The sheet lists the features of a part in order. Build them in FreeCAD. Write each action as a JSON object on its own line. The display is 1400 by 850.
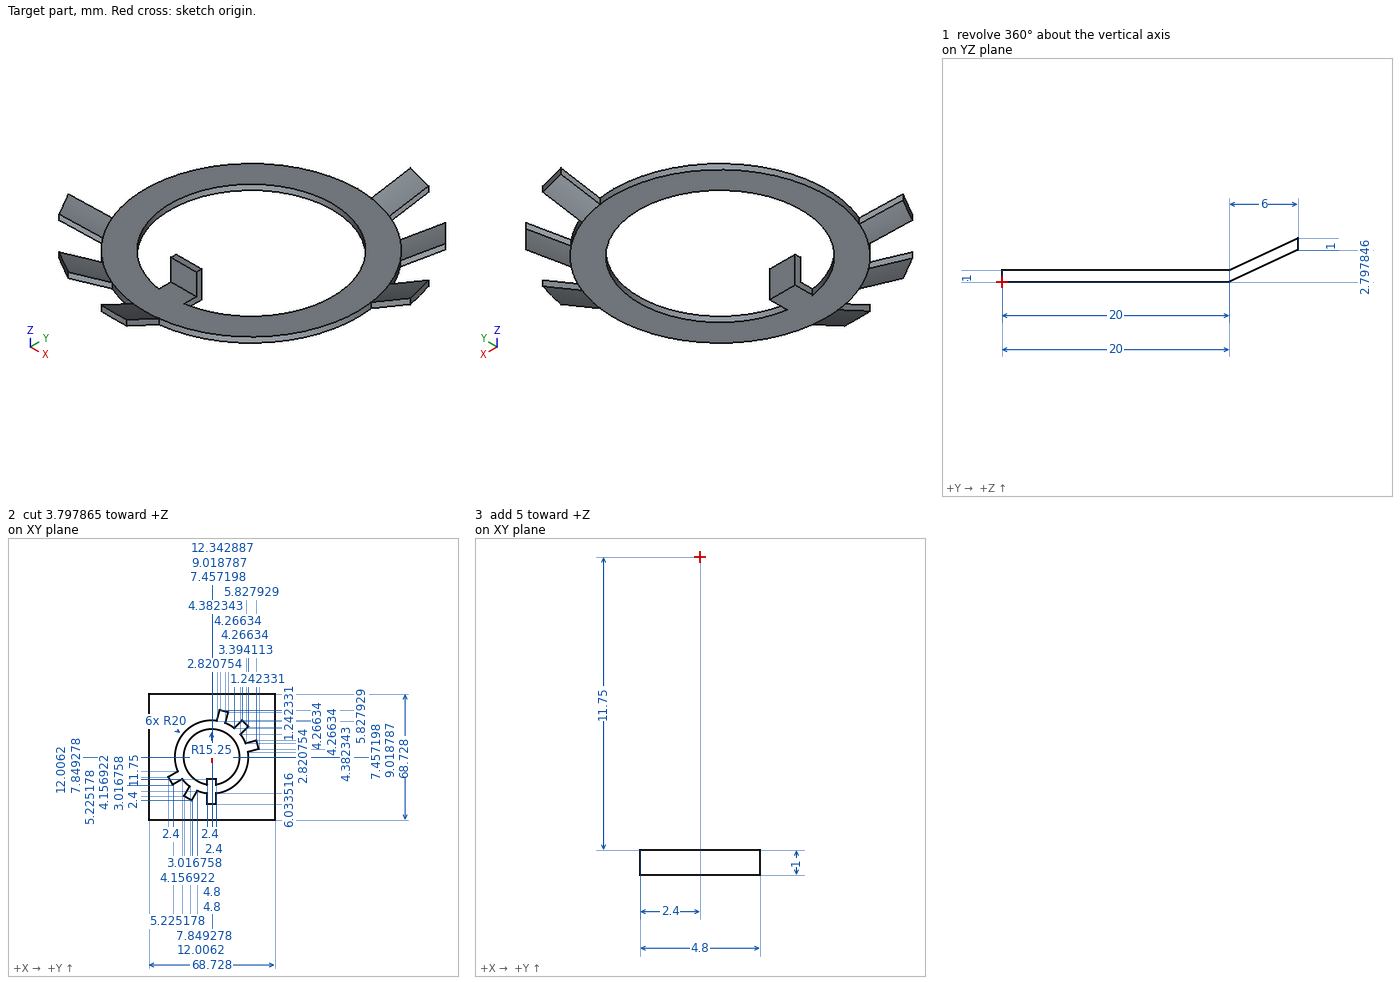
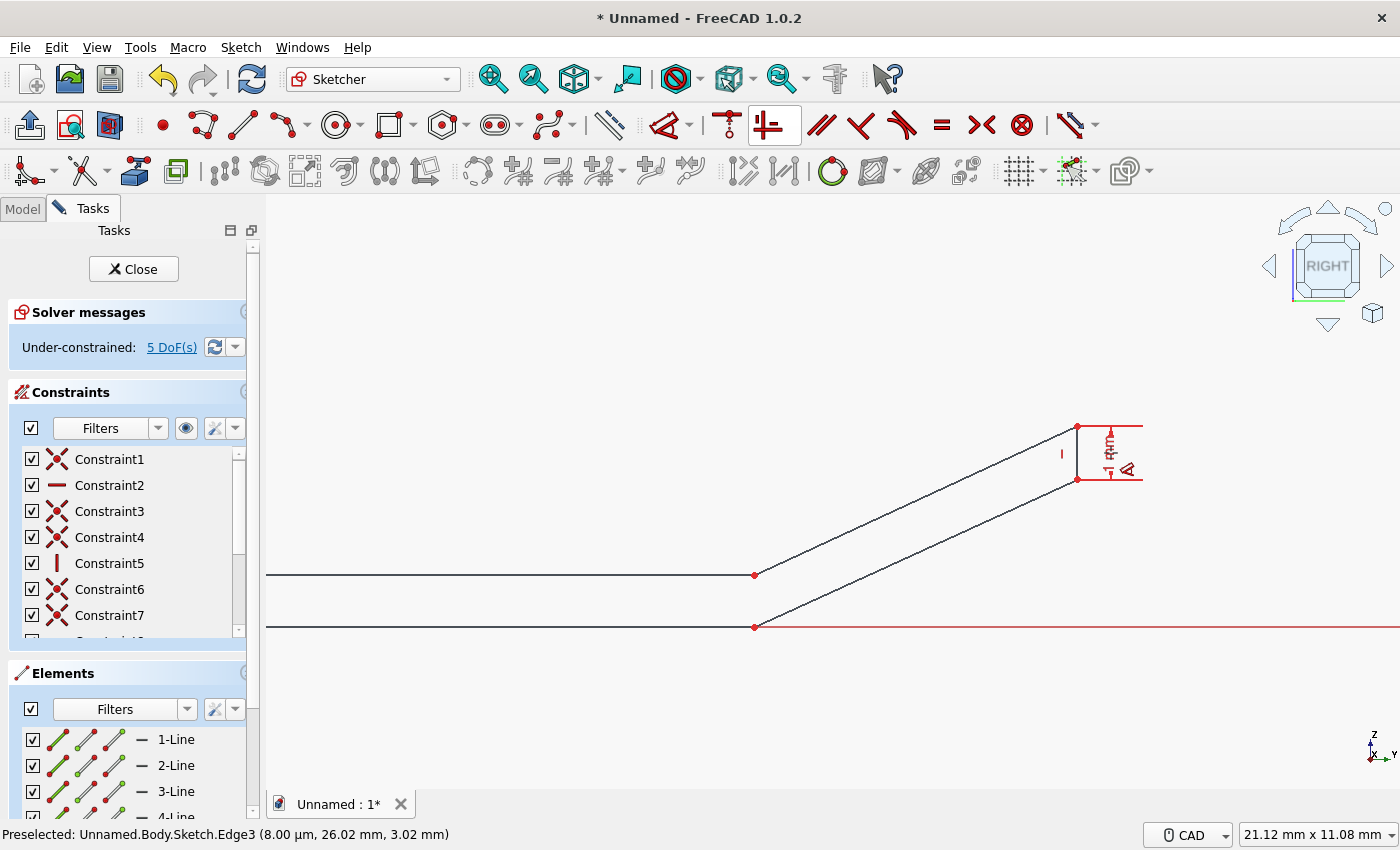
{"action": "scroll", "coordinate": [1080, 464], "scroll_direction": "down", "scroll_amount": 4}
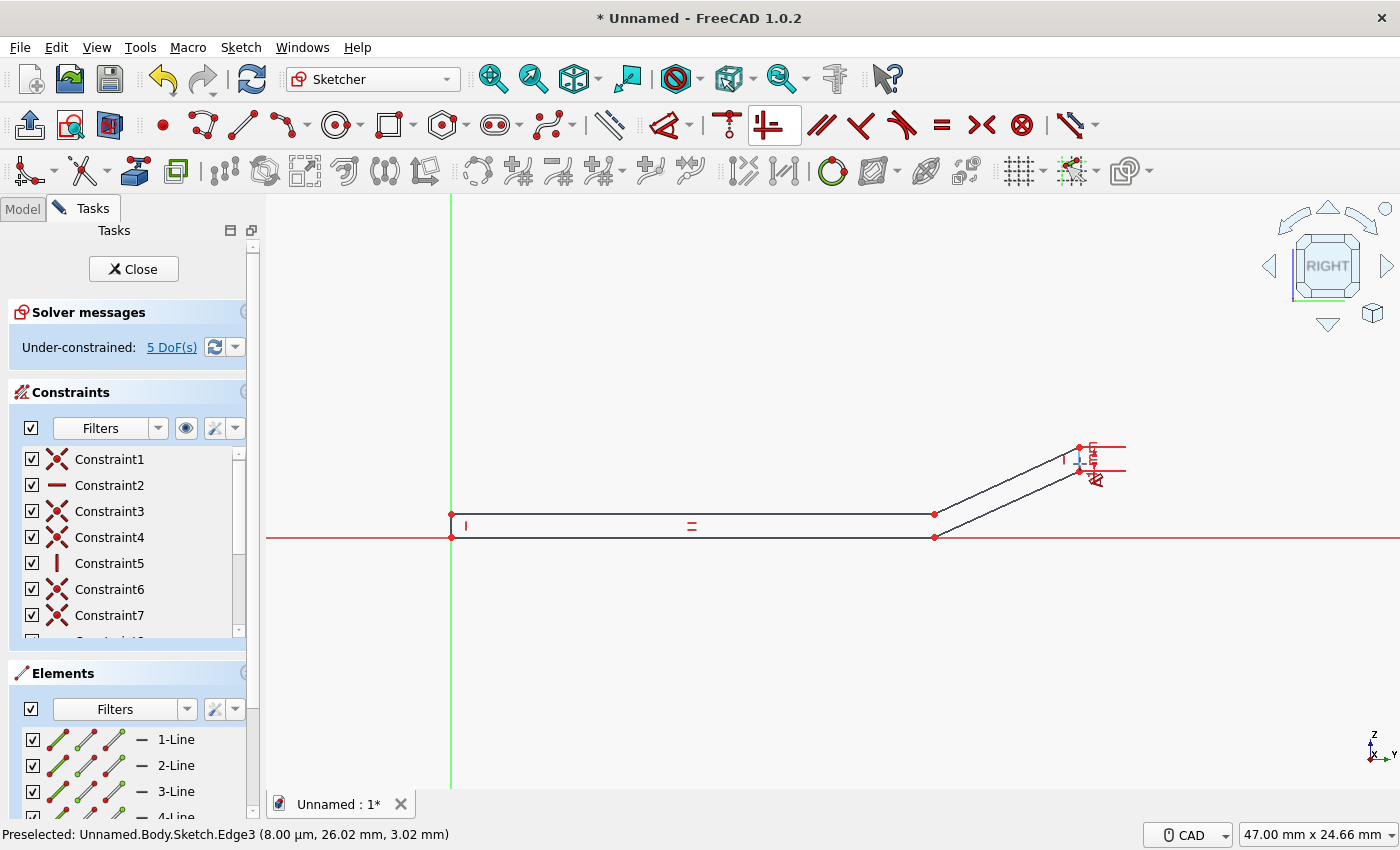
{"action": "scroll", "coordinate": [451, 521], "scroll_direction": "up", "scroll_amount": 4}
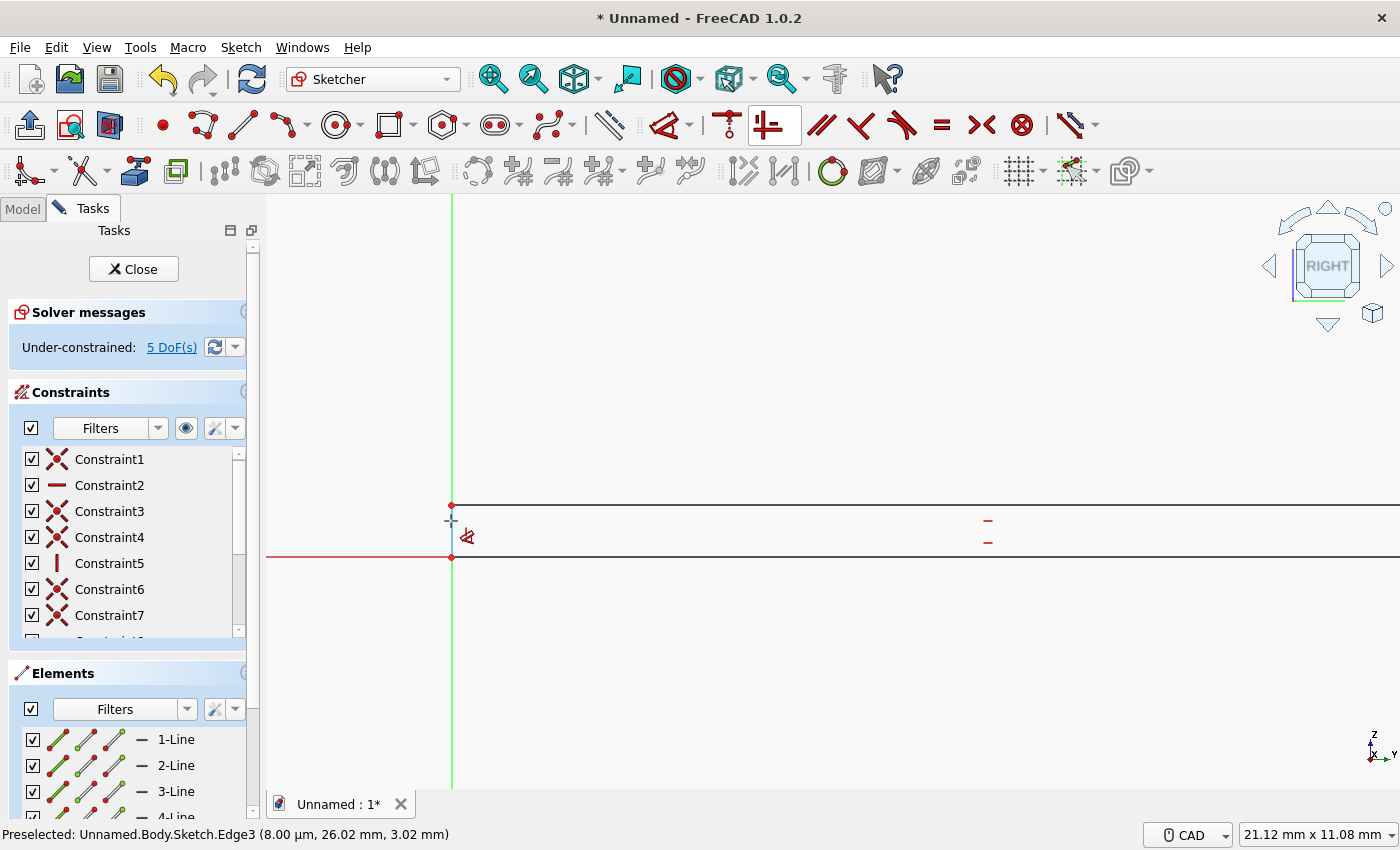
{"action": "left_click", "coordinate": [452, 521]}
{"action": "left_click", "coordinate": [418, 531]}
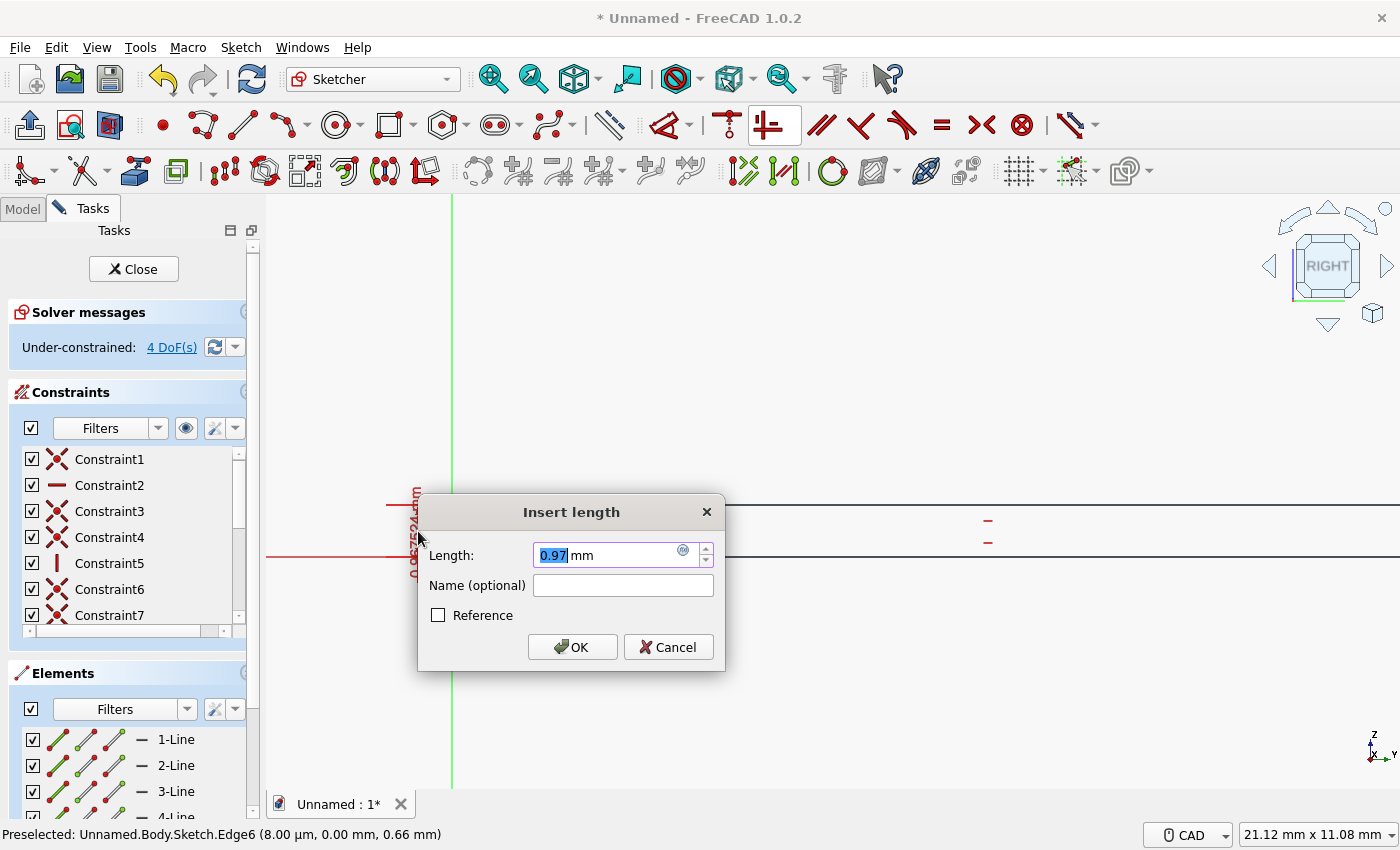
{"action": "type", "text": "1"}
{"action": "key", "text": "Return"}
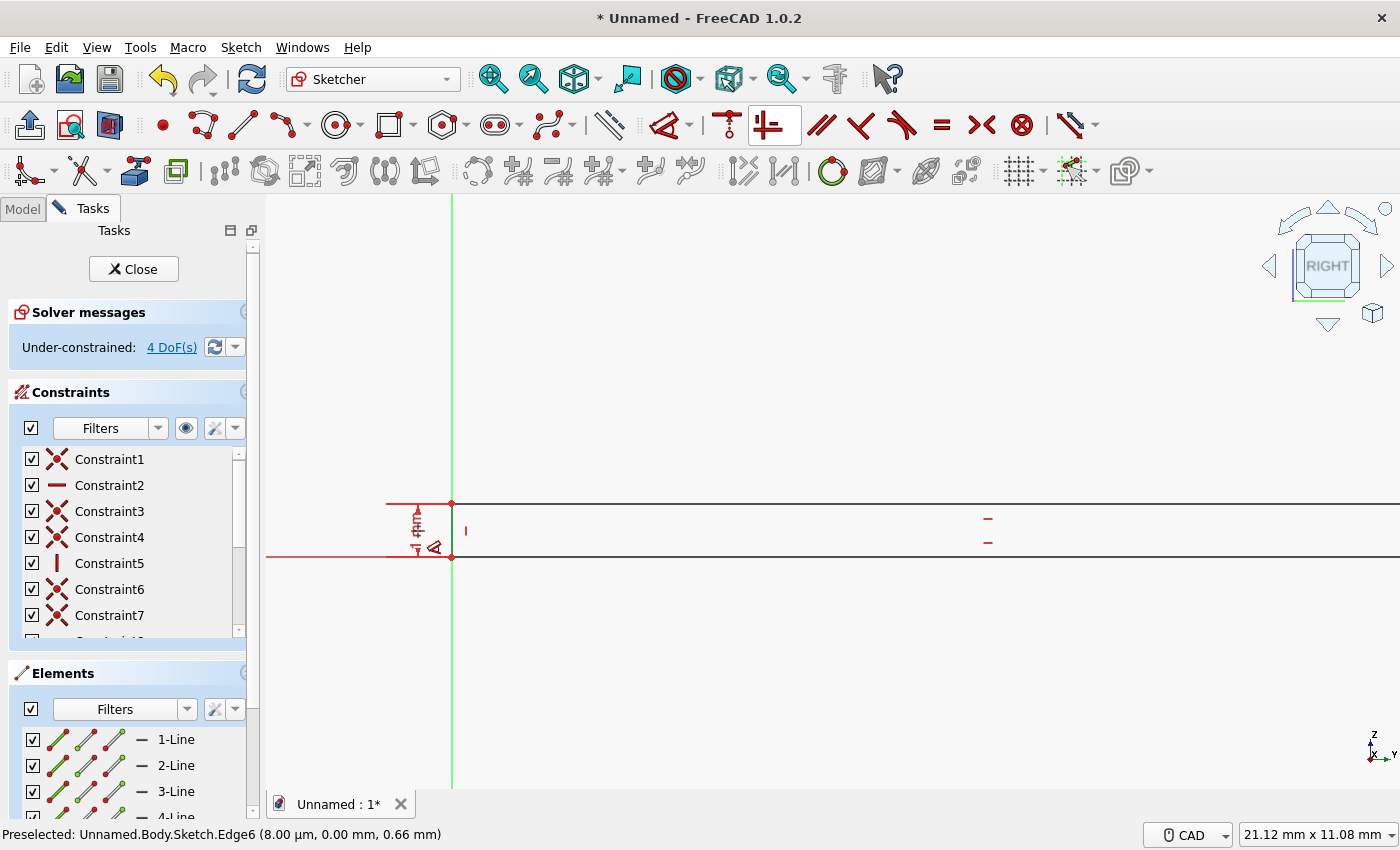
{"action": "left_click", "coordinate": [774, 557]}
{"action": "left_click", "coordinate": [843, 591]}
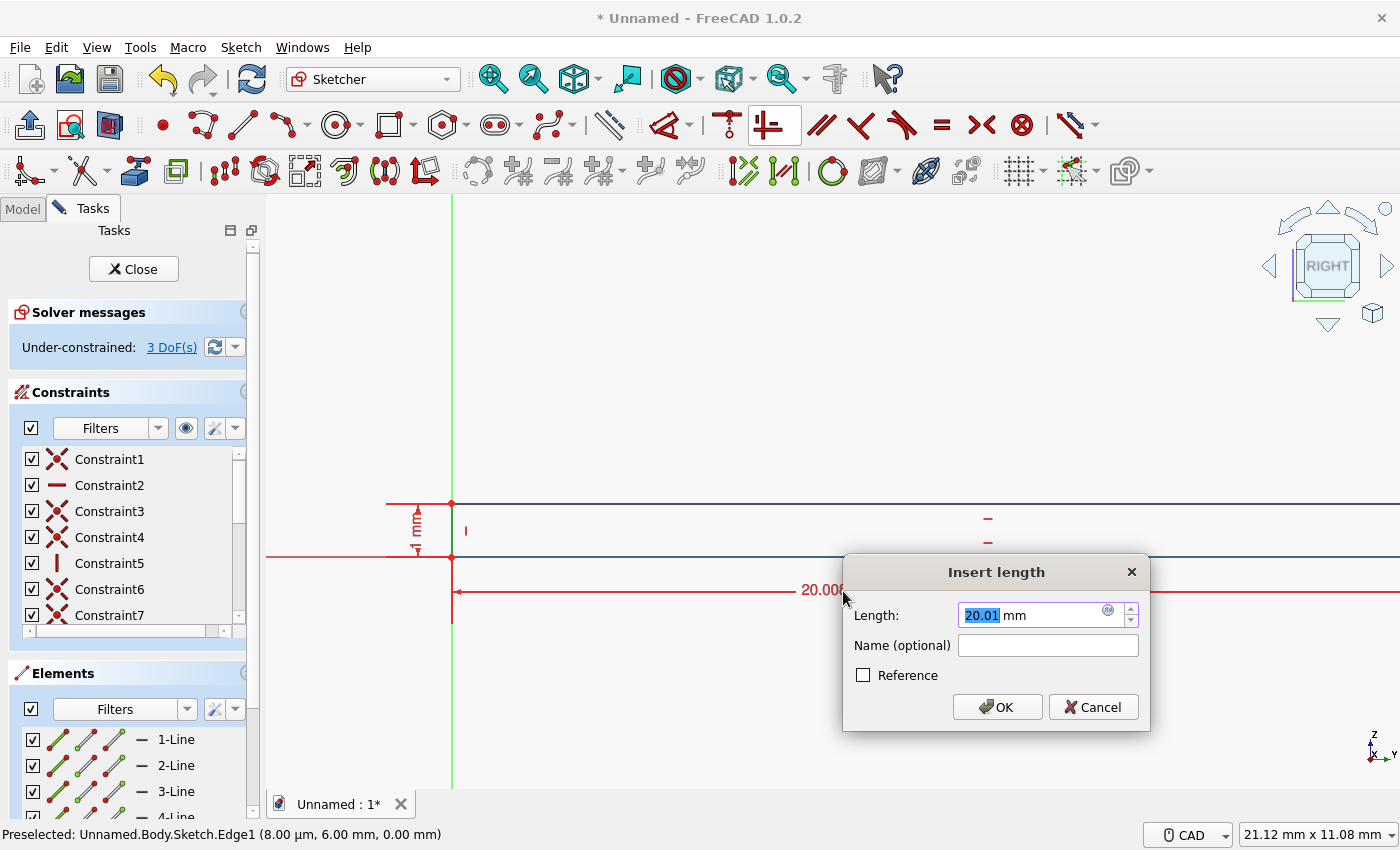
{"action": "type", "text": "20"}
{"action": "key", "text": "Return"}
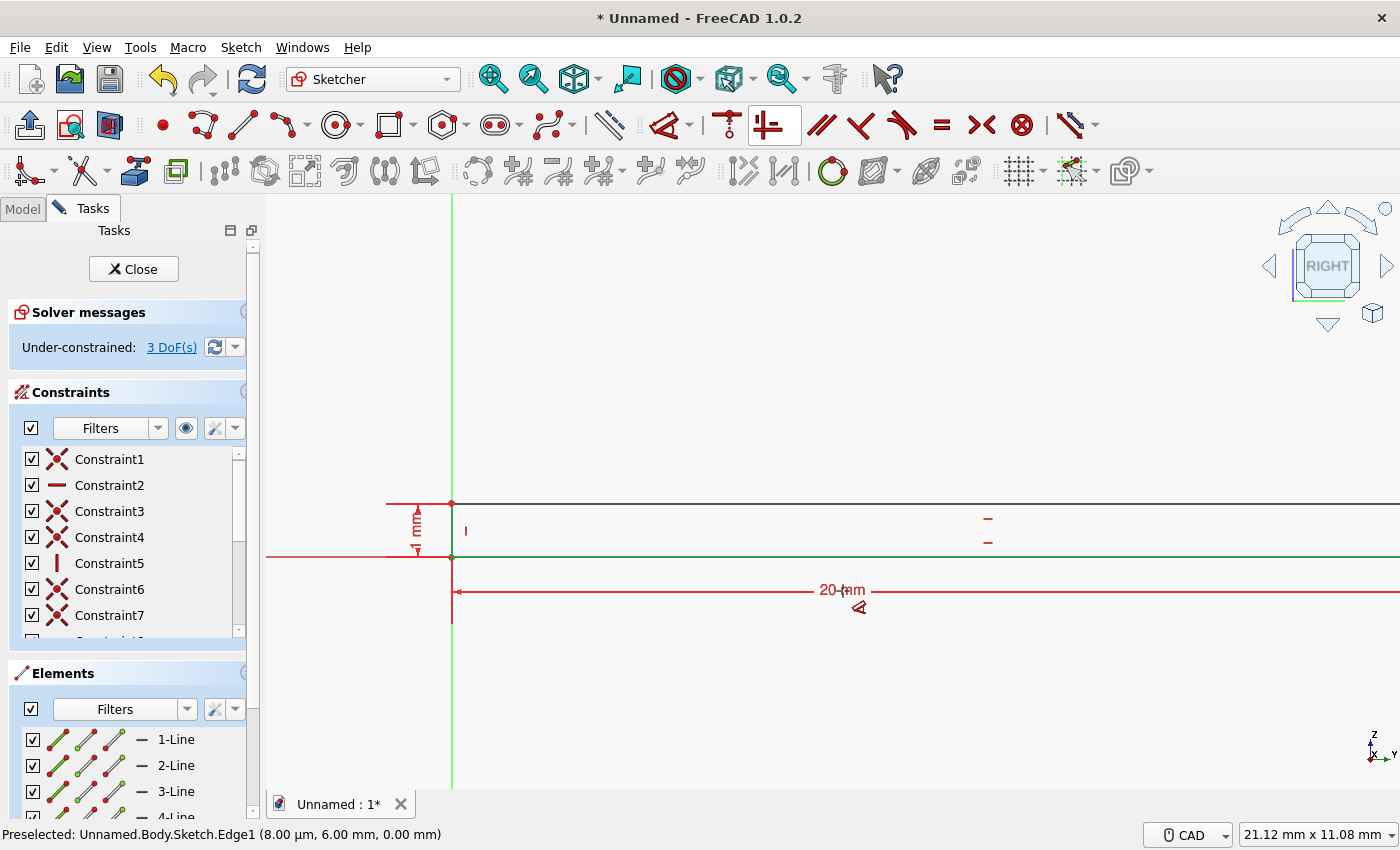
{"action": "left_click", "coordinate": [1204, 504]}
{"action": "left_click", "coordinate": [843, 538]}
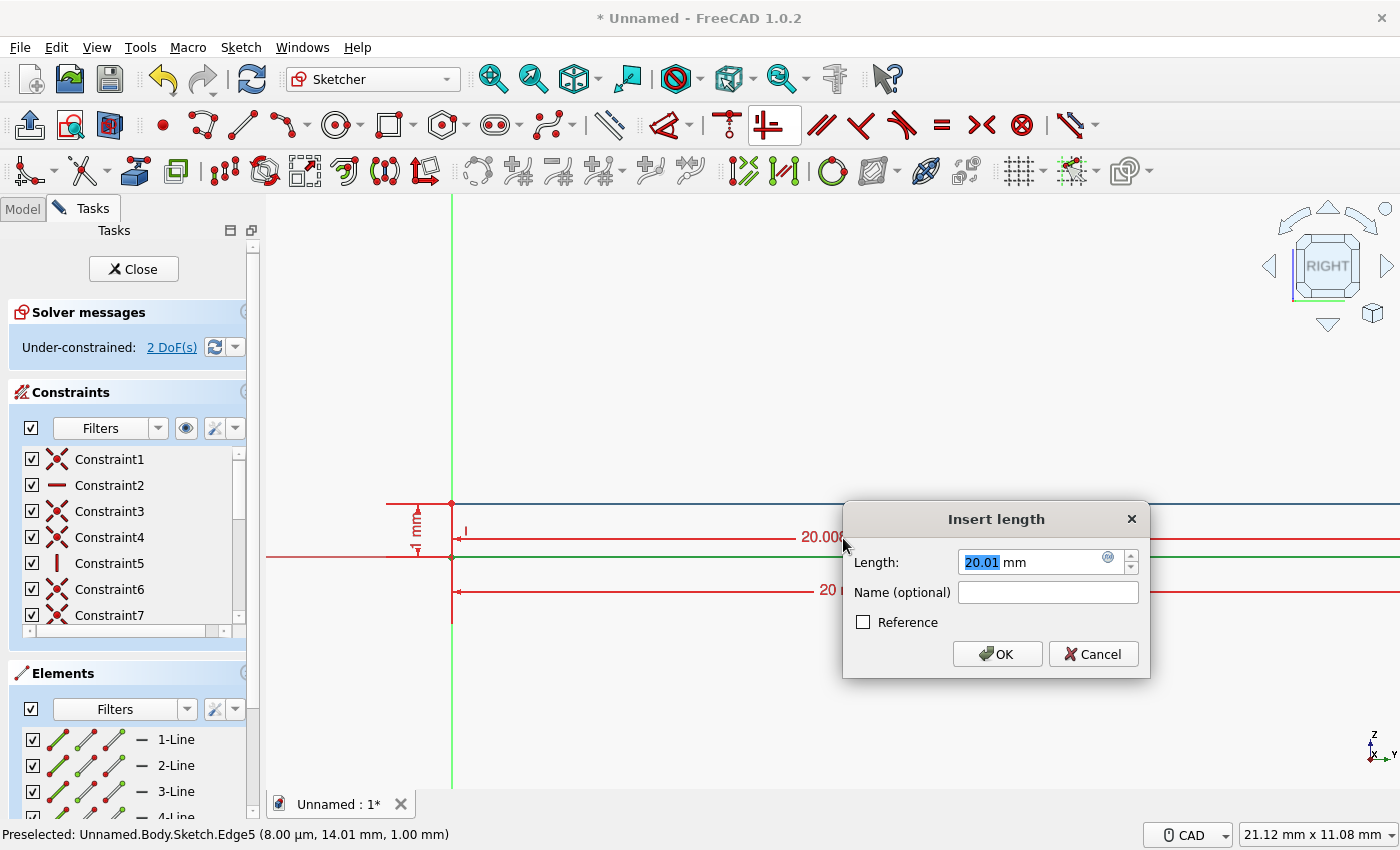
{"action": "type", "text": "20"}
{"action": "key", "text": "Return"}